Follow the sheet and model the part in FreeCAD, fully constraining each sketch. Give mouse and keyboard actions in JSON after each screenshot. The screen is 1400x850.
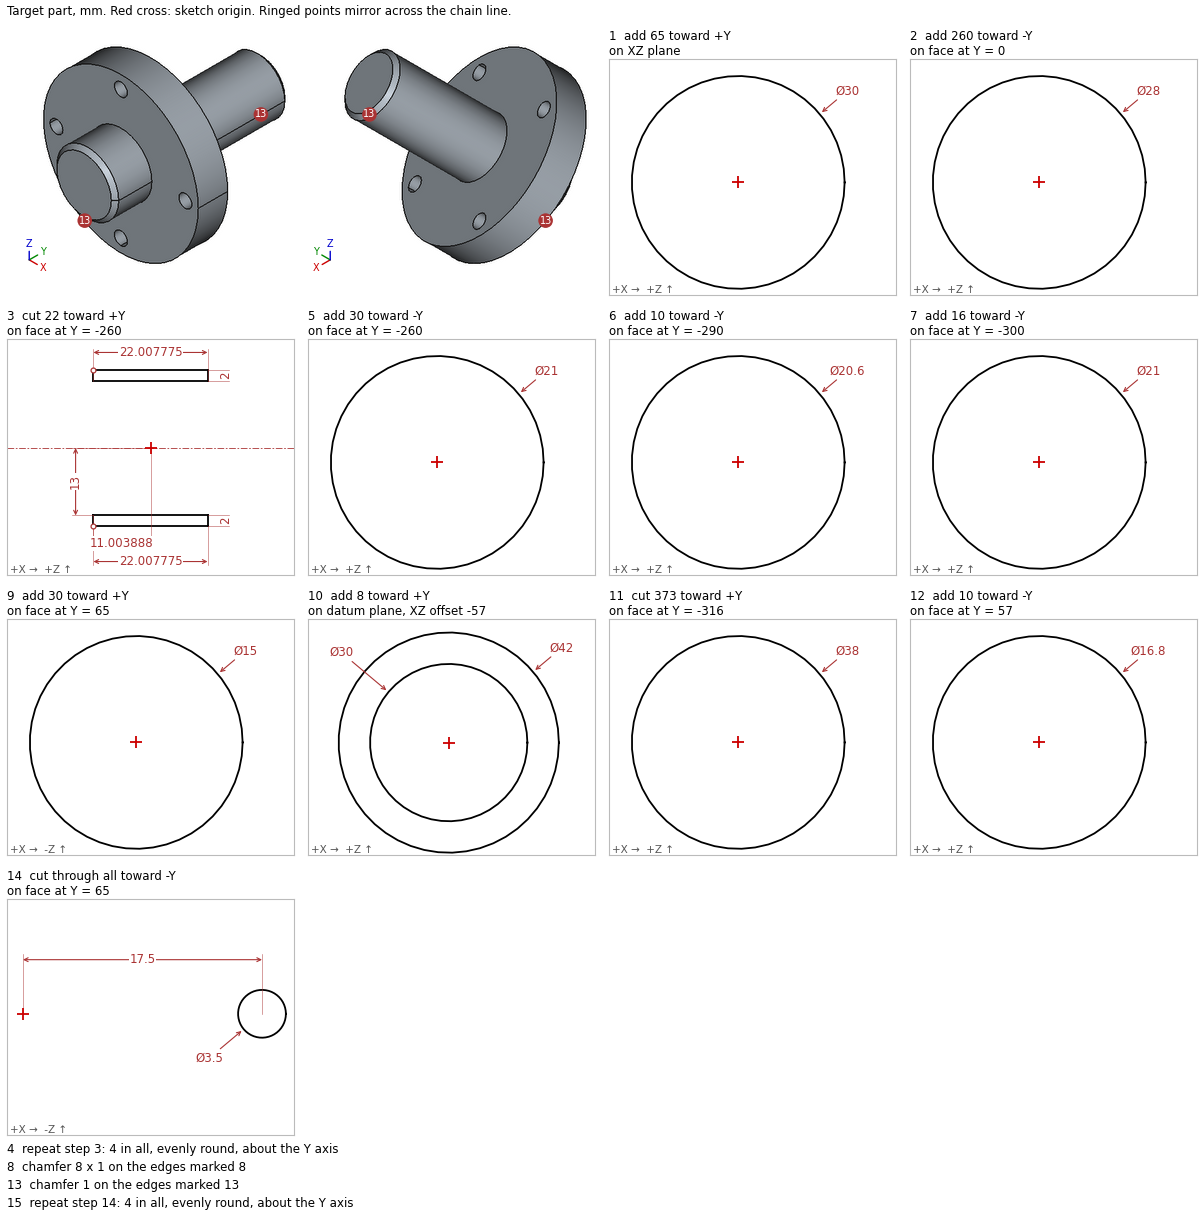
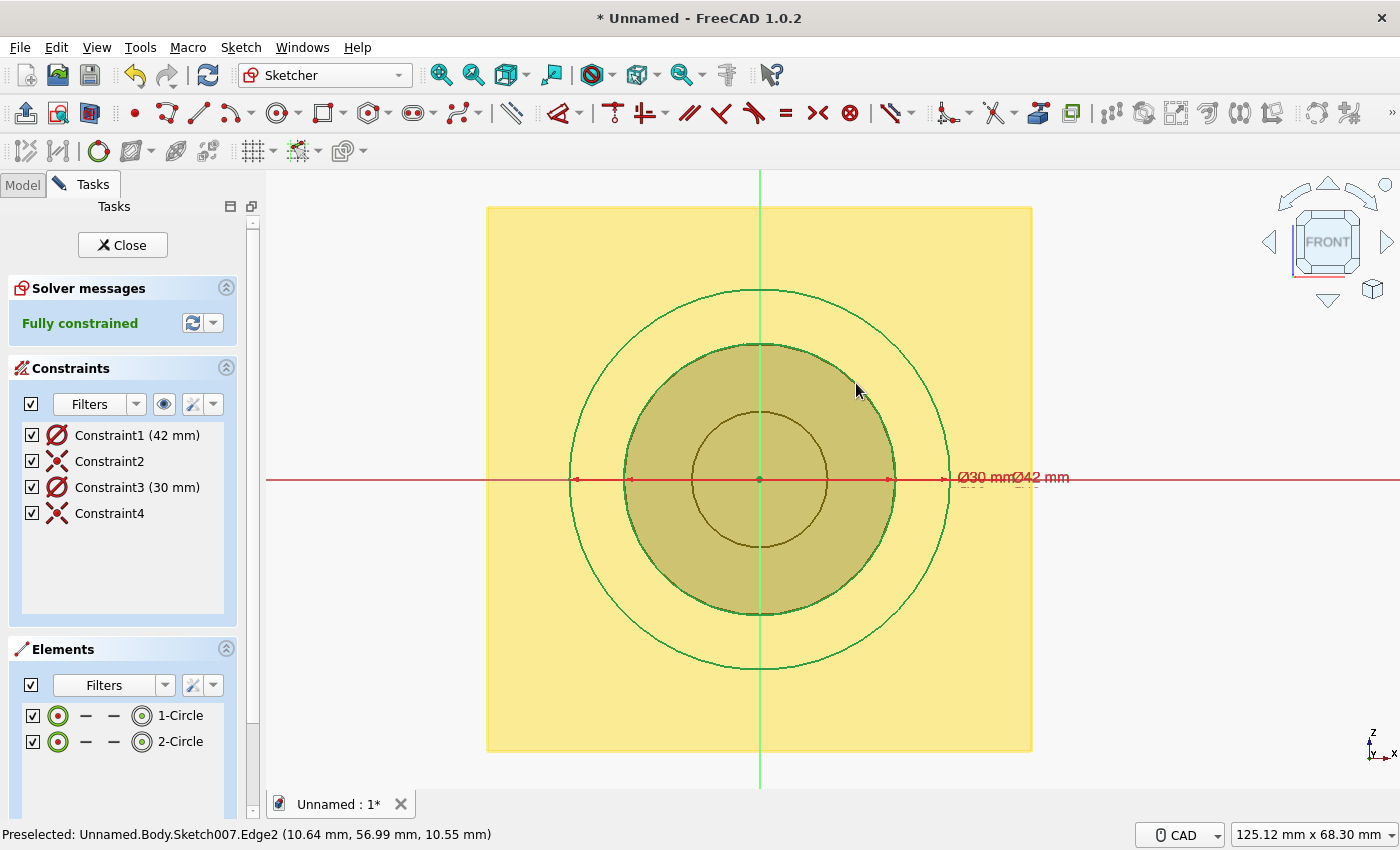
{"action": "left_click", "coordinate": [123, 245]}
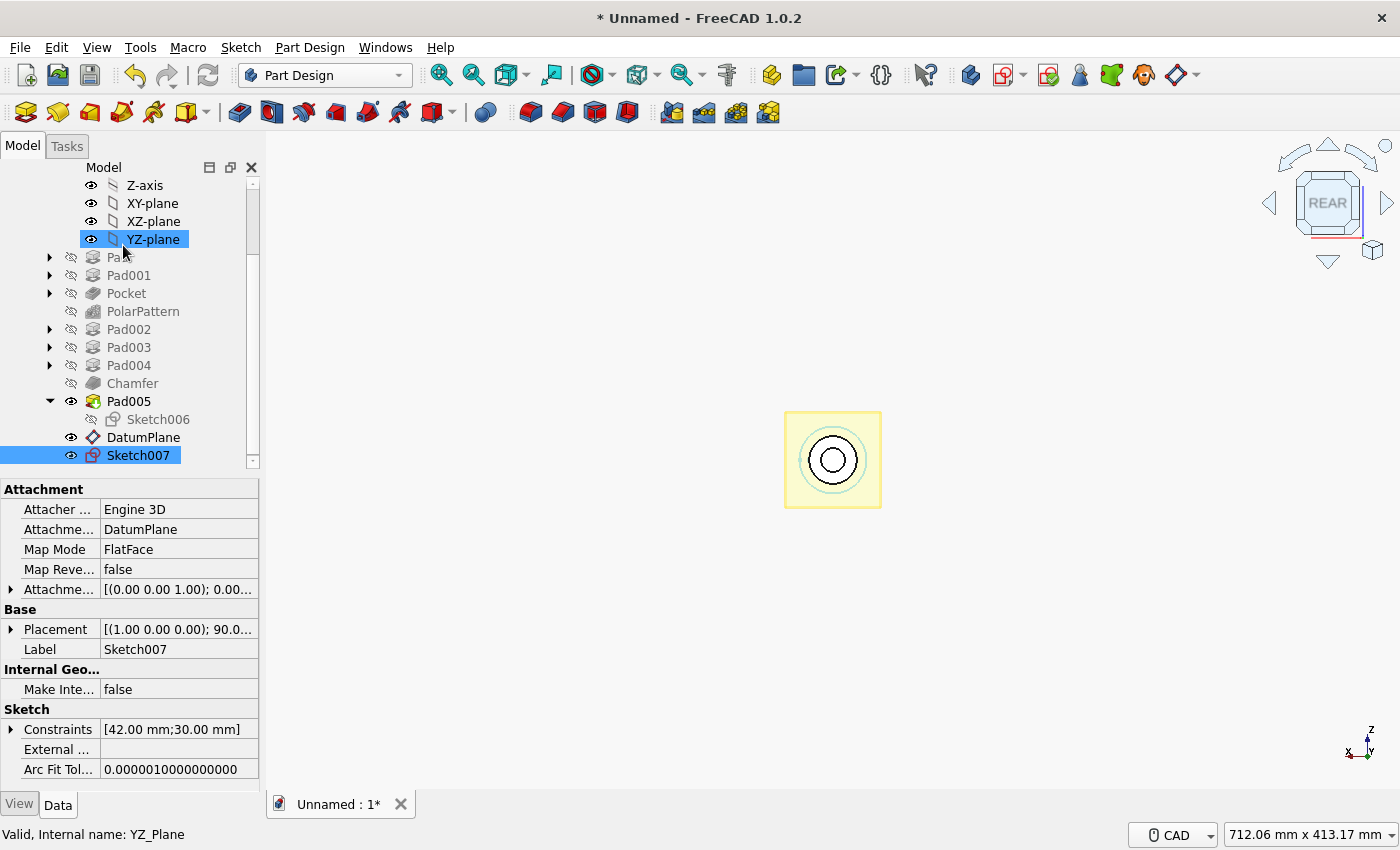
{"action": "left_click", "coordinate": [26, 112]}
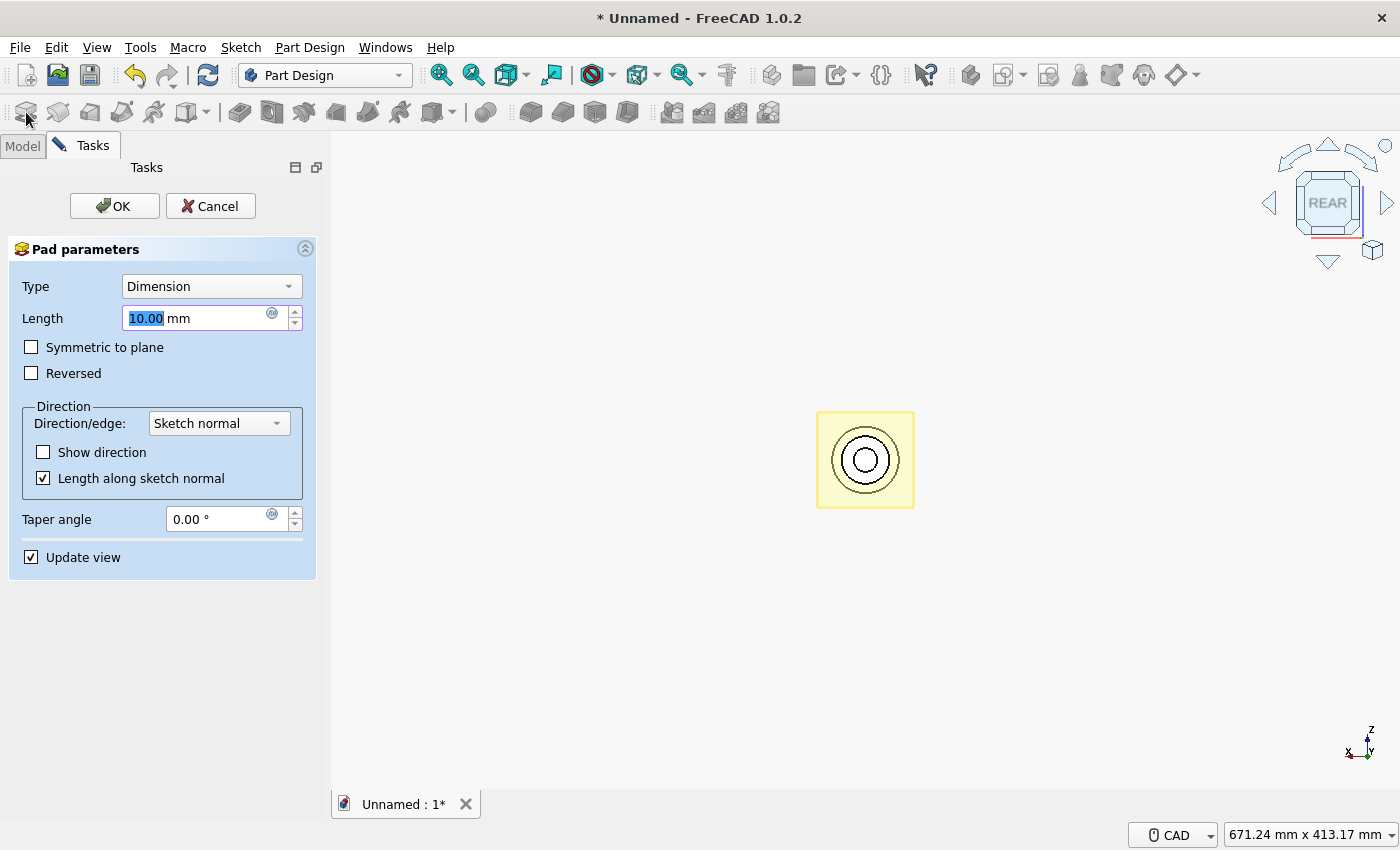
{"action": "type", "text": "8"}
{"action": "key", "text": "Tab"}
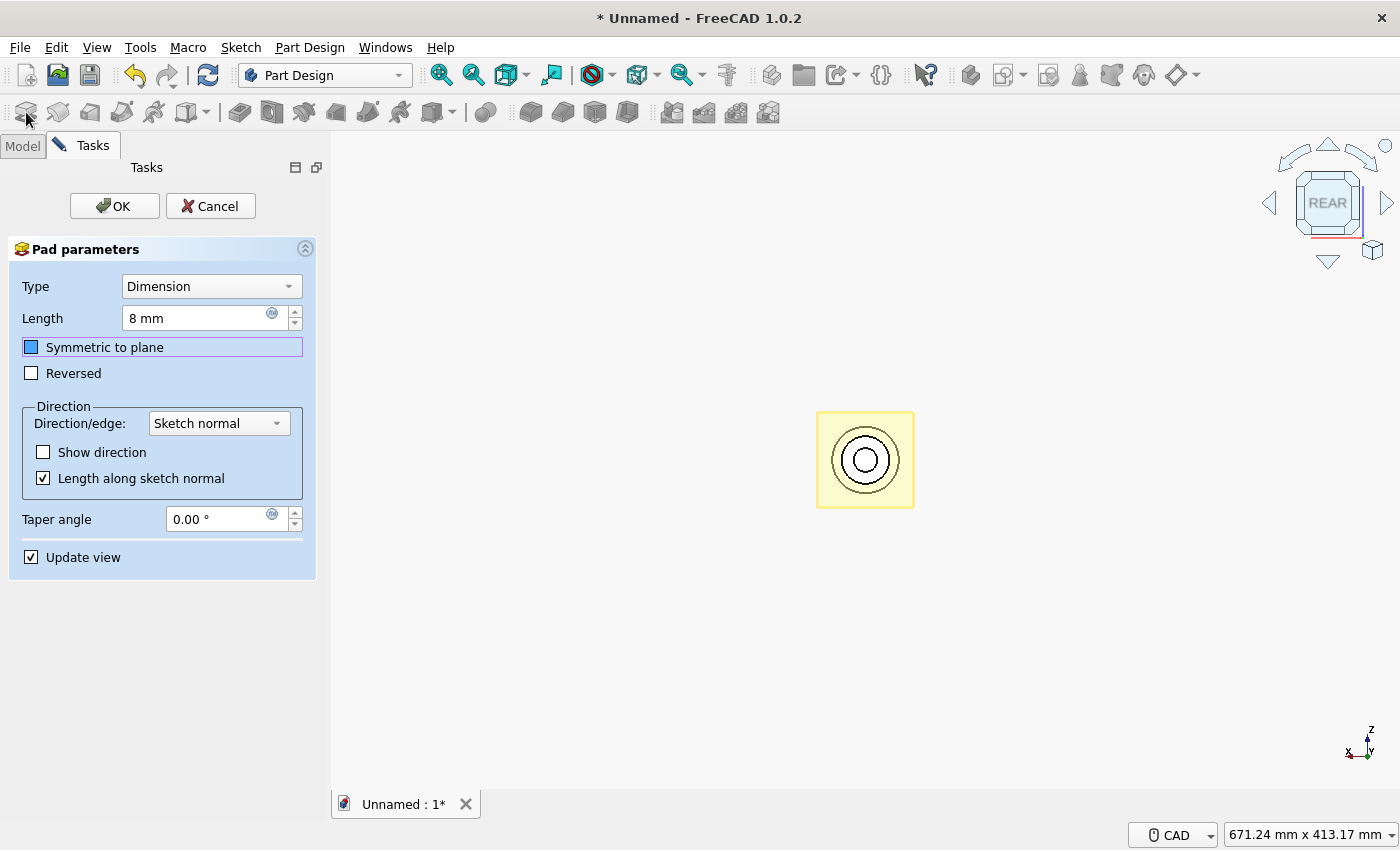
{"action": "left_click", "coordinate": [30, 373]}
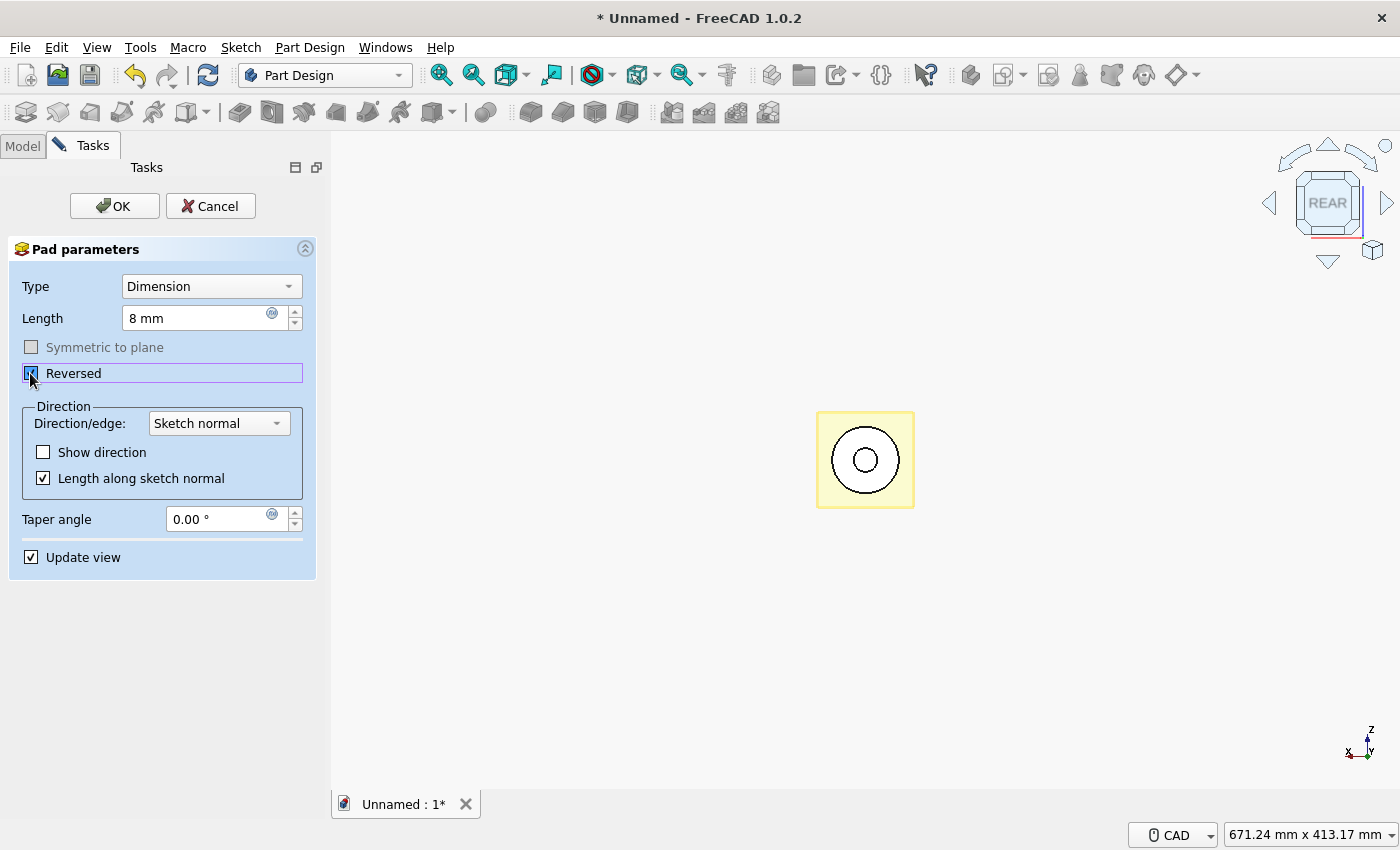
{"action": "left_click", "coordinate": [115, 206]}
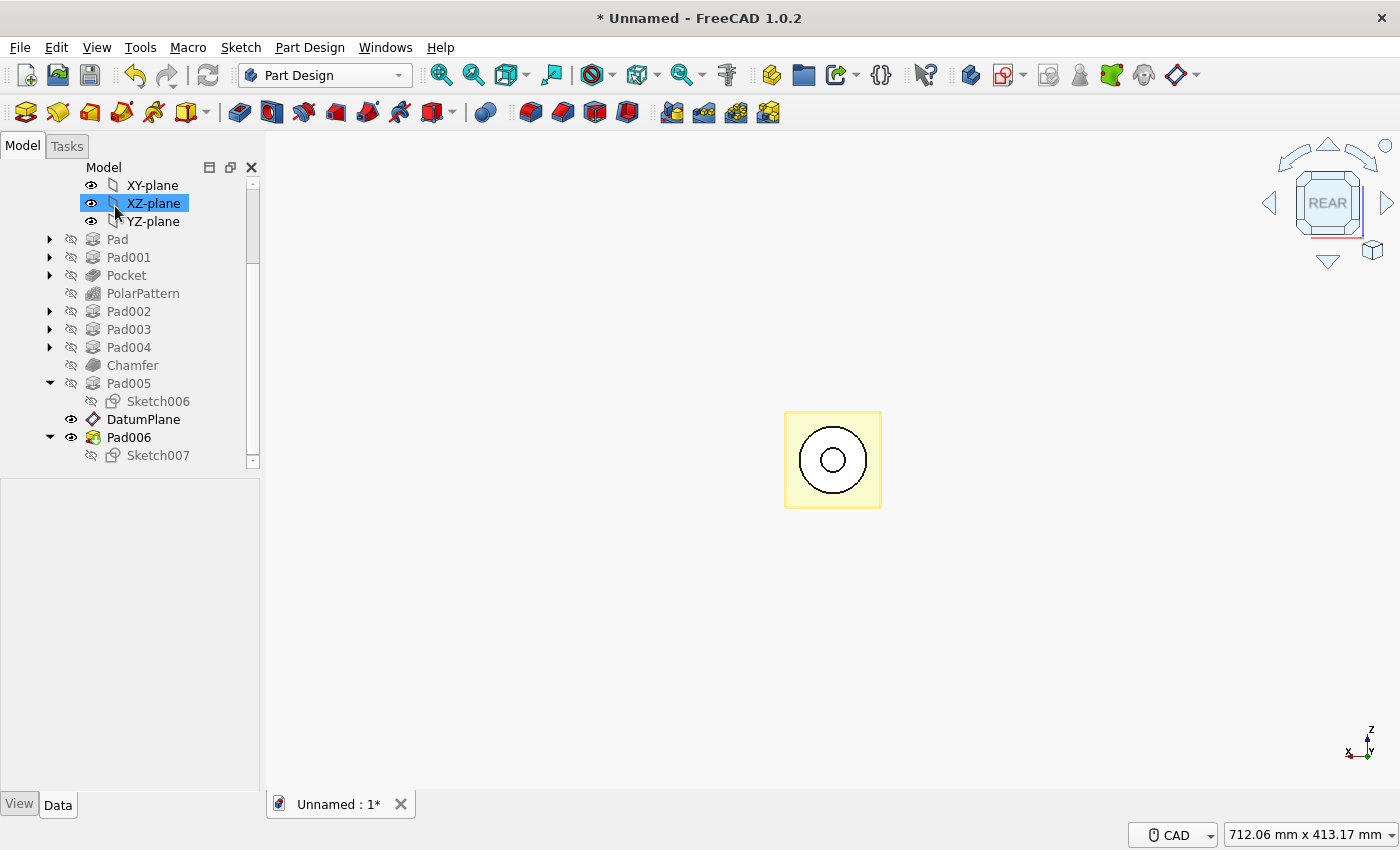
{"action": "left_click", "coordinate": [116, 419]}
{"action": "key", "text": "space"}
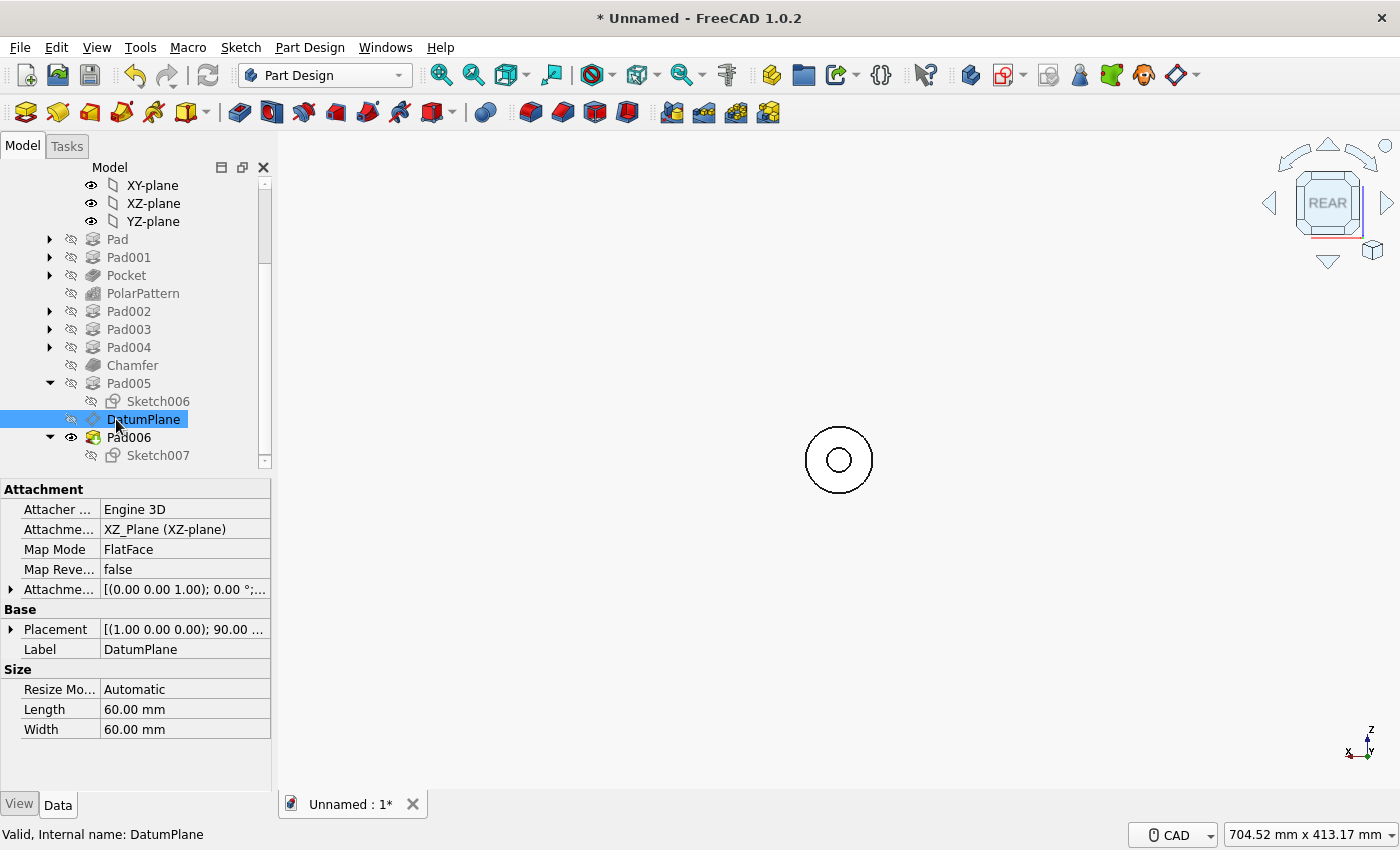
{"action": "left_click", "coordinate": [442, 76]}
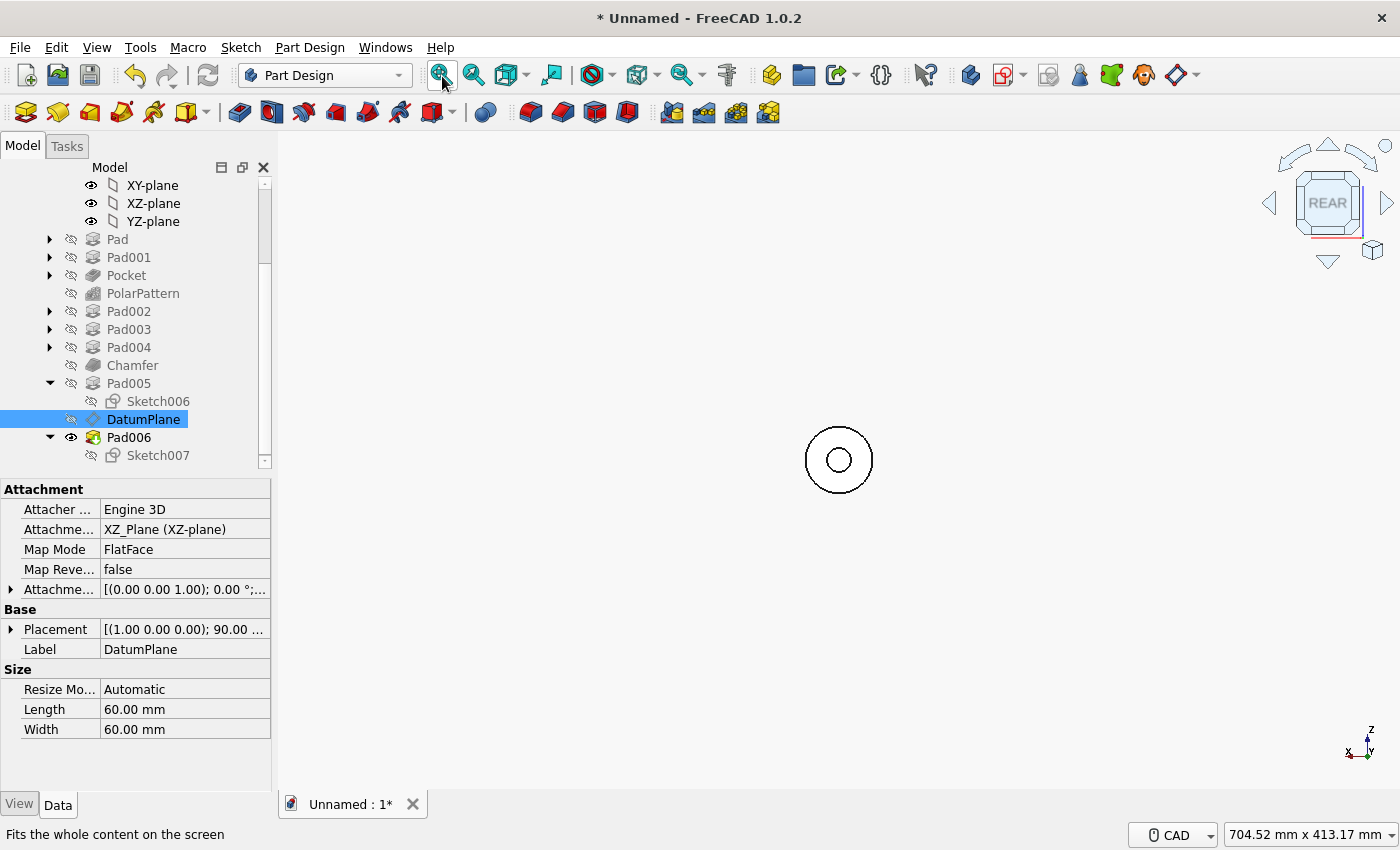
{"action": "key", "text": "0"}